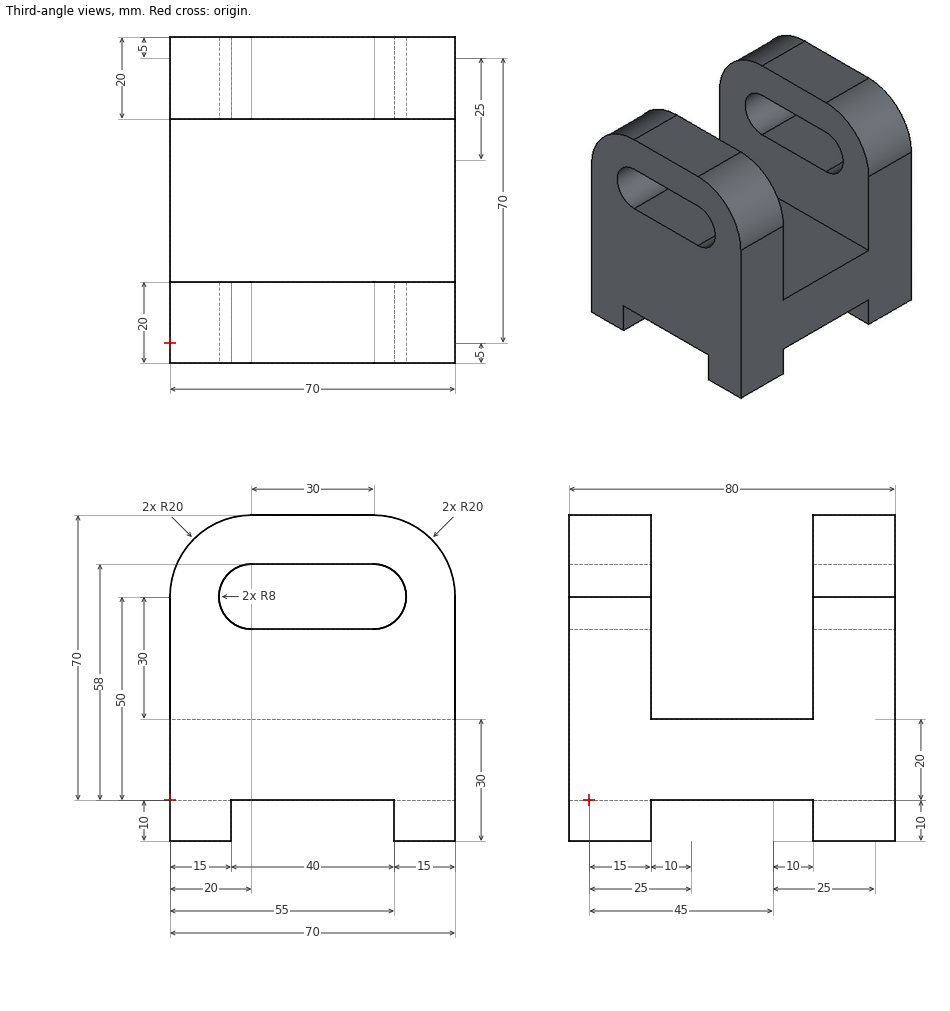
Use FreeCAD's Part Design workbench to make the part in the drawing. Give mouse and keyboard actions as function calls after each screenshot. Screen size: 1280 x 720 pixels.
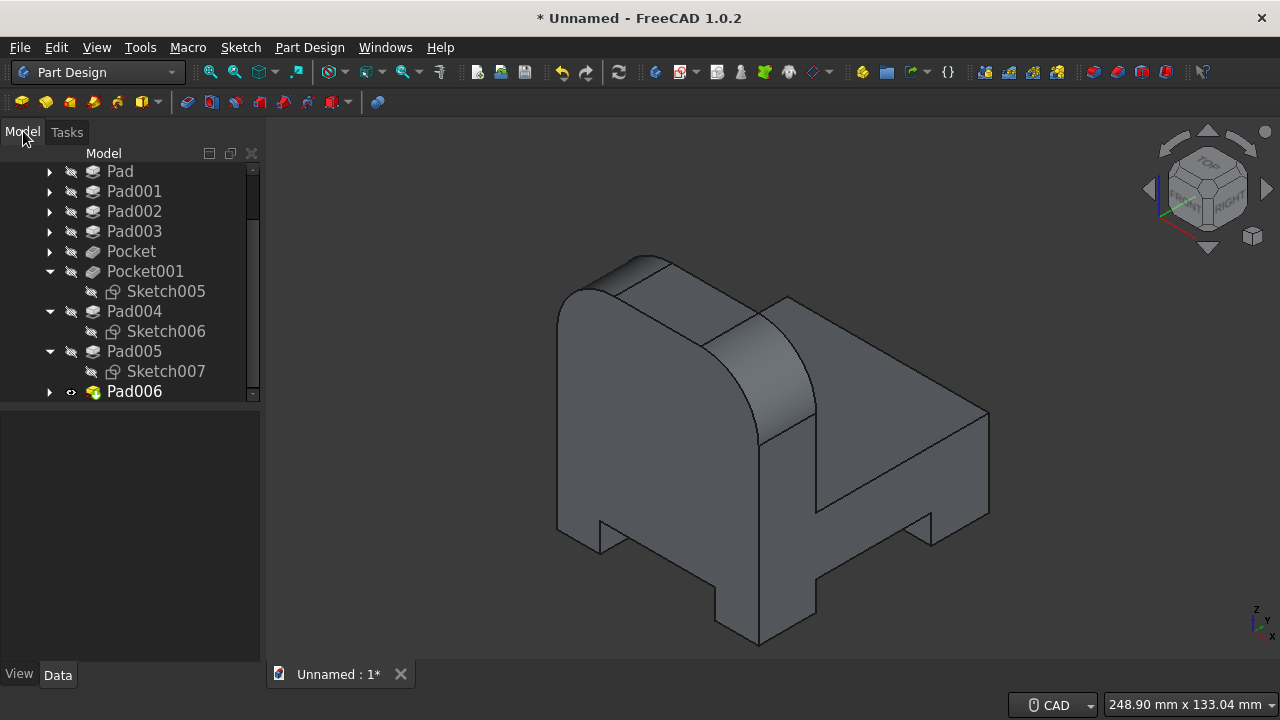
scroll(140, 287, down, 3)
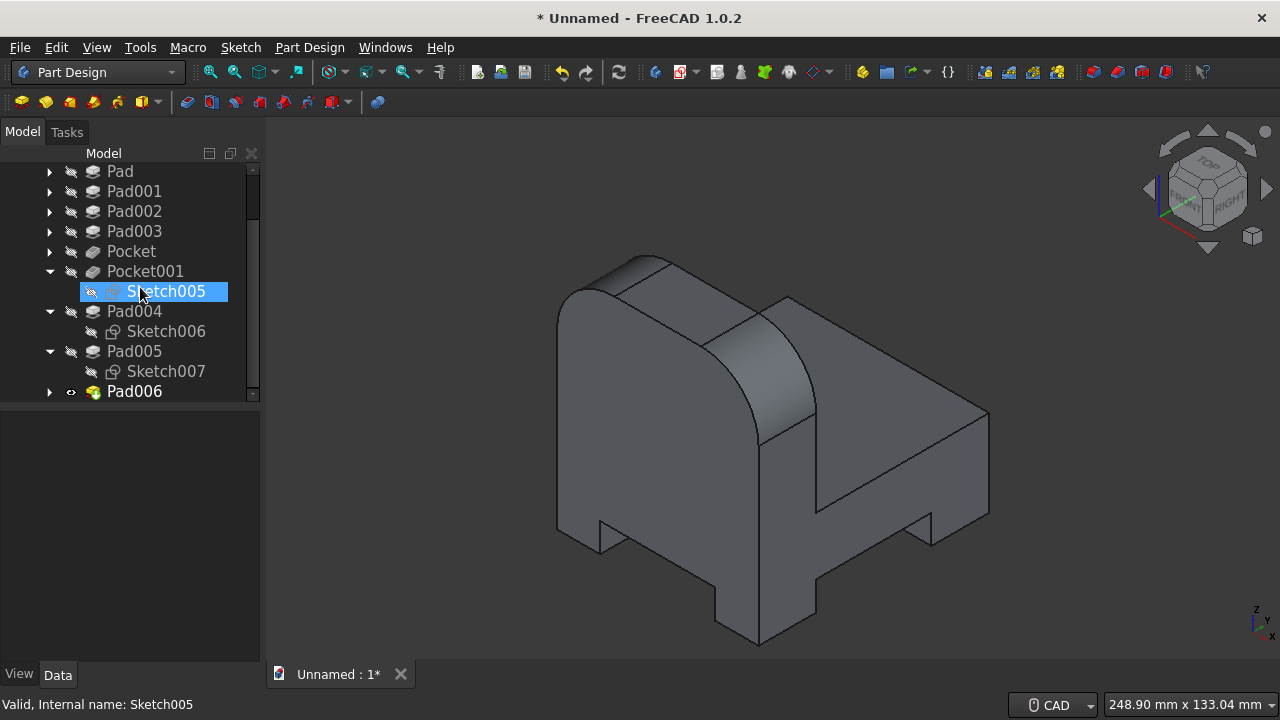
scroll(140, 287, up, 15)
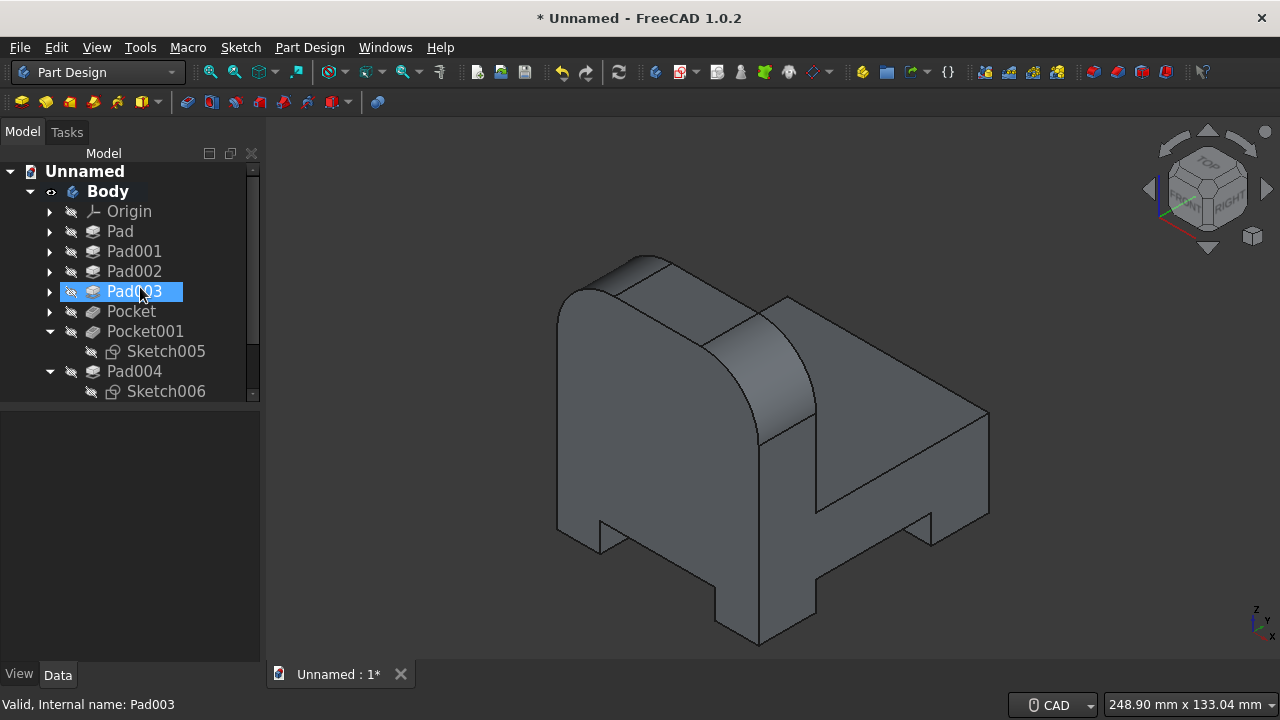
click(50, 212)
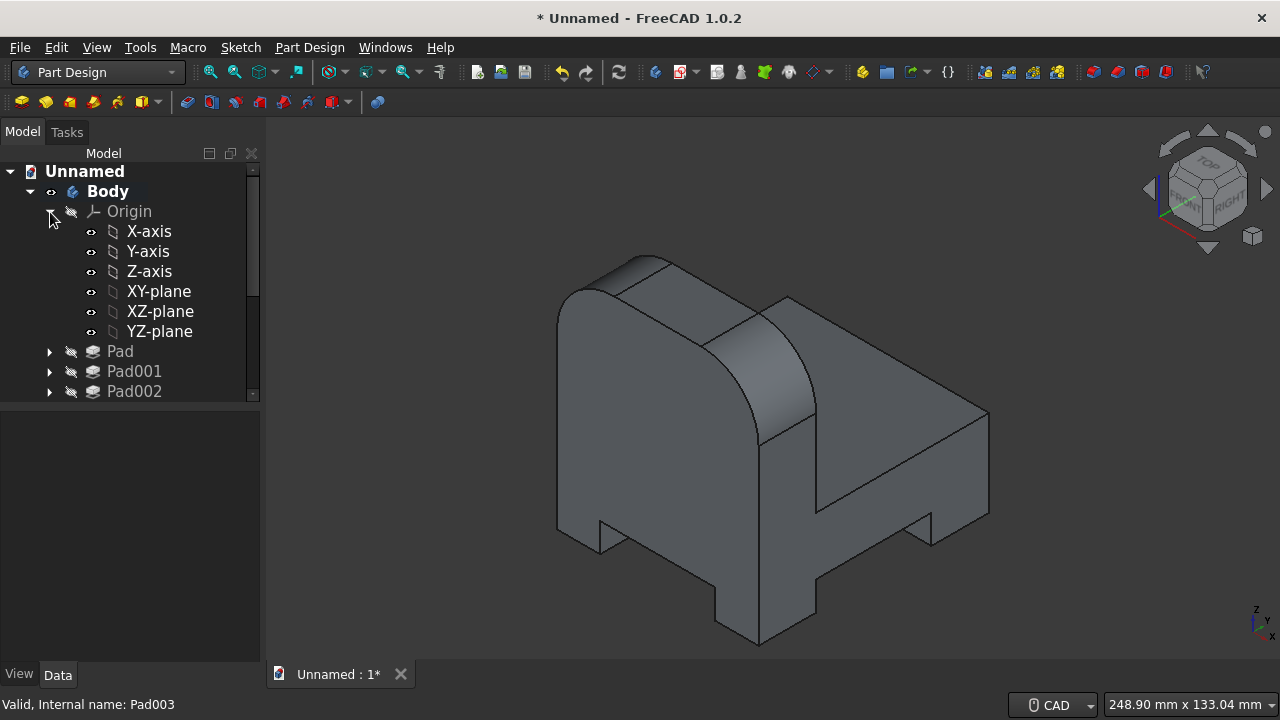
click(136, 312)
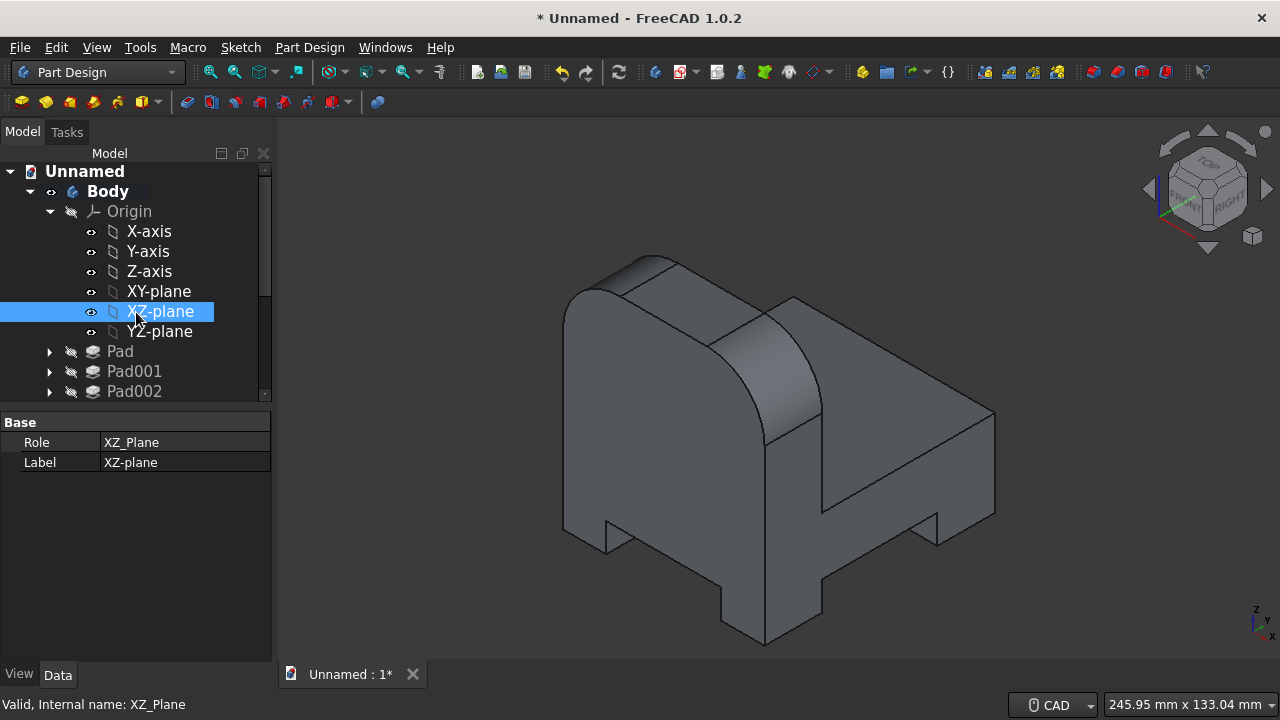
click(814, 72)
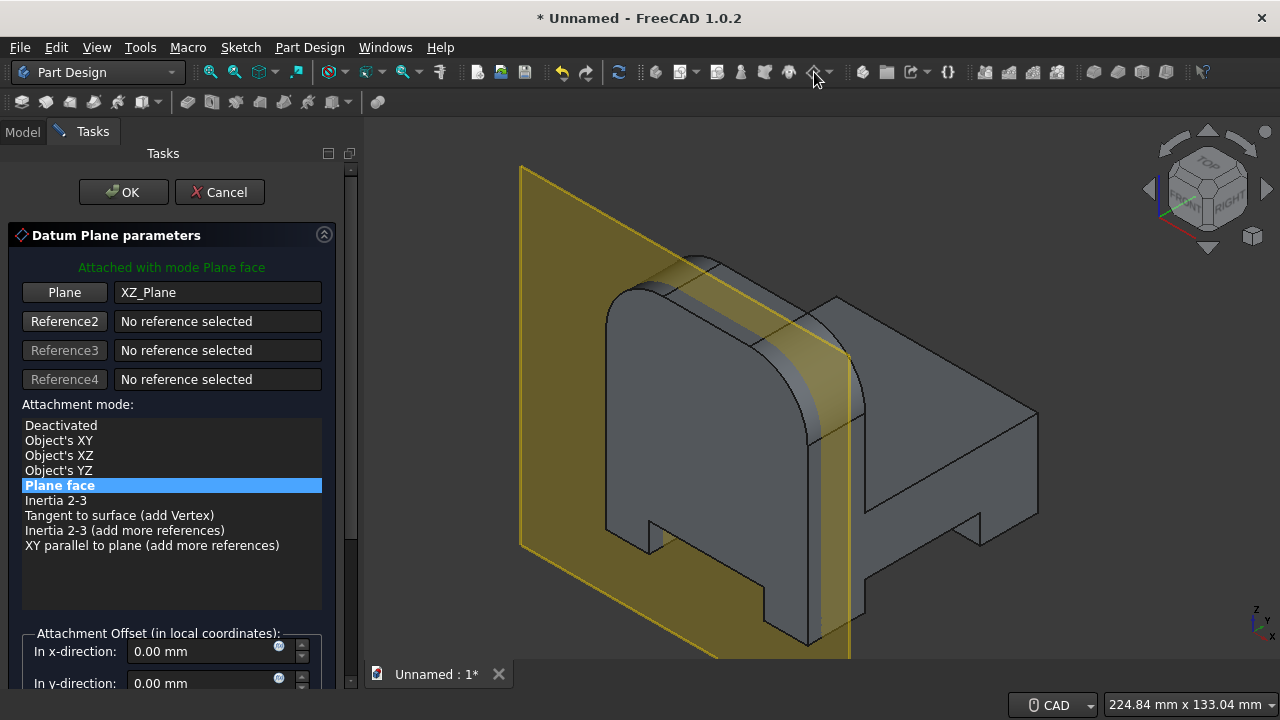
scroll(351, 426, down, 2)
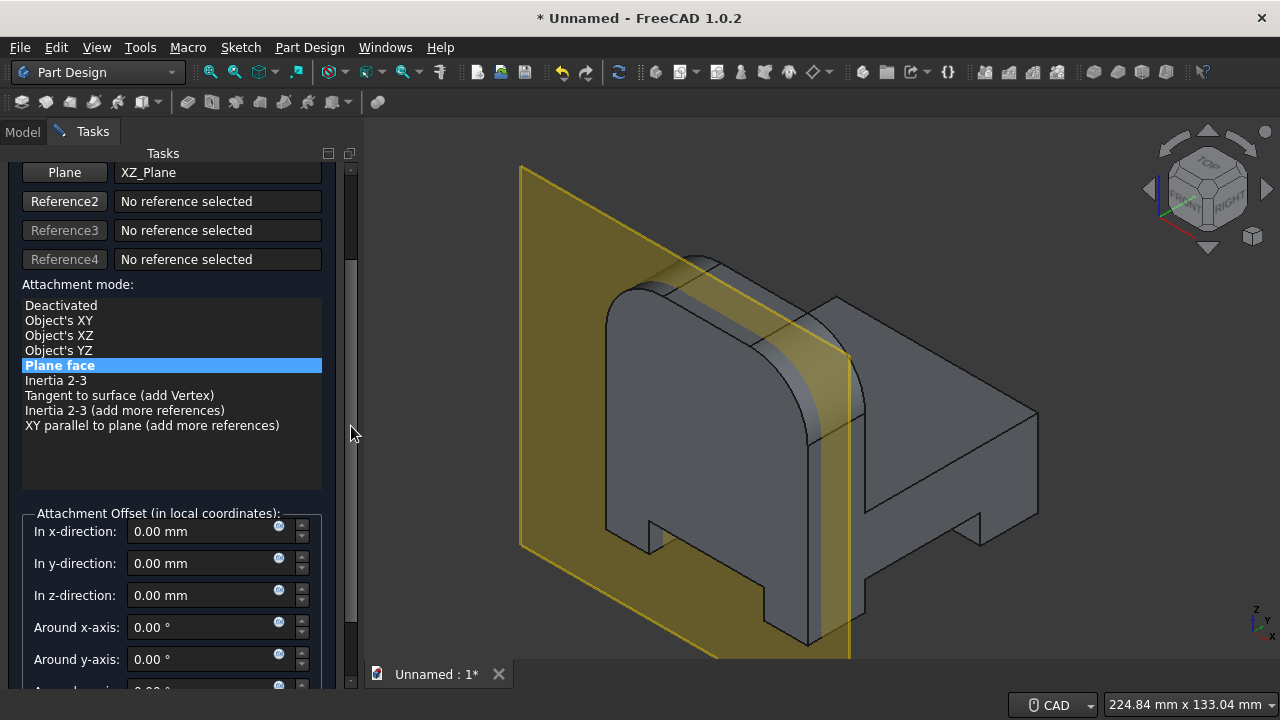
triple_click(210, 595)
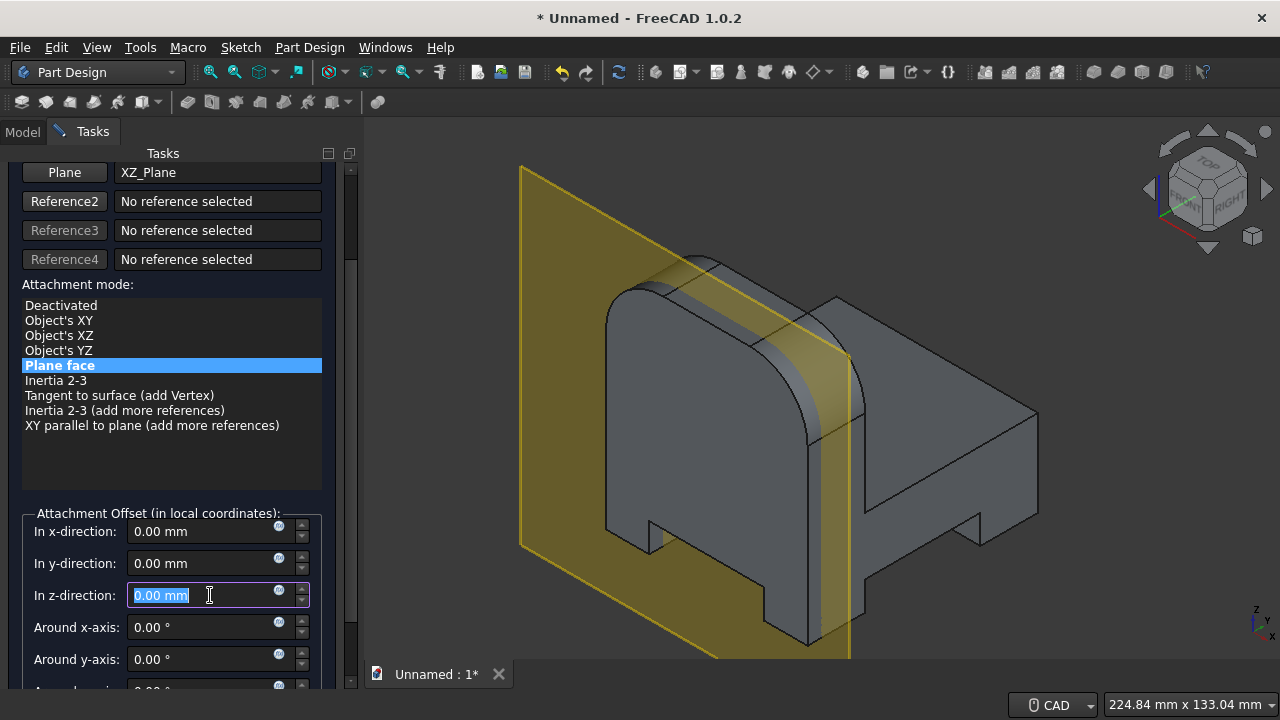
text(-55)
key(Tab)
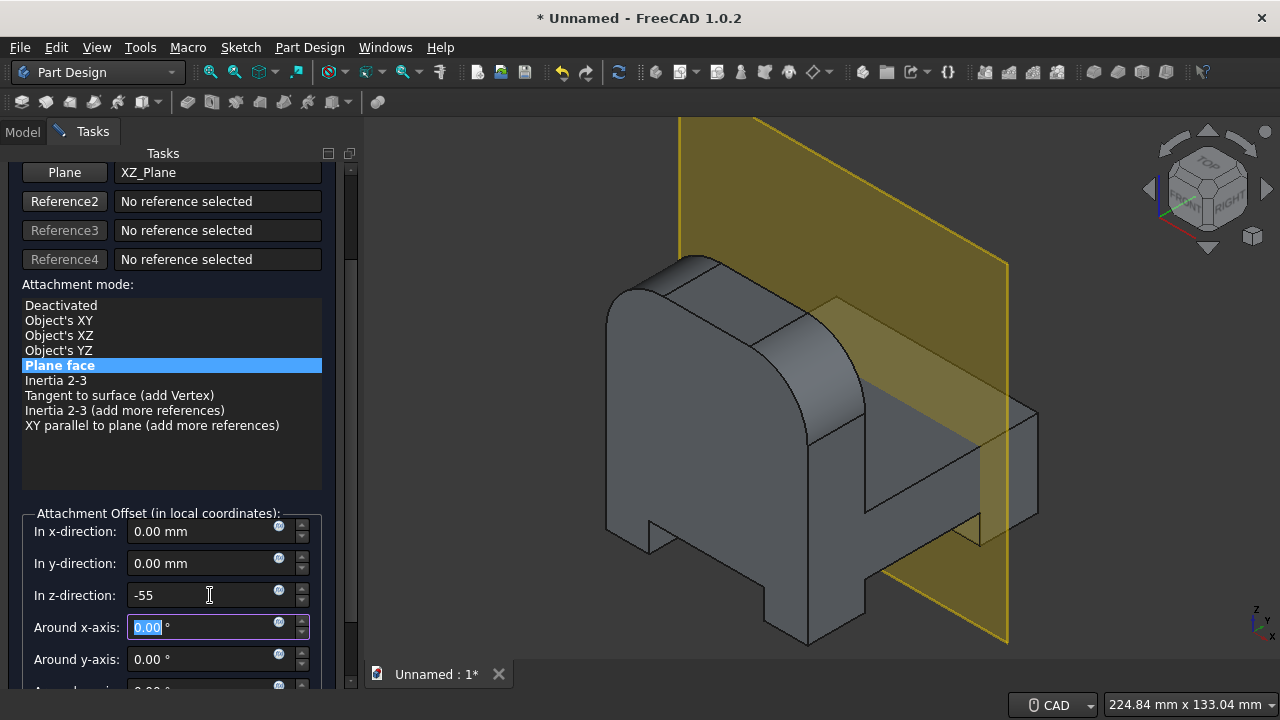
scroll(351, 426, up, 3)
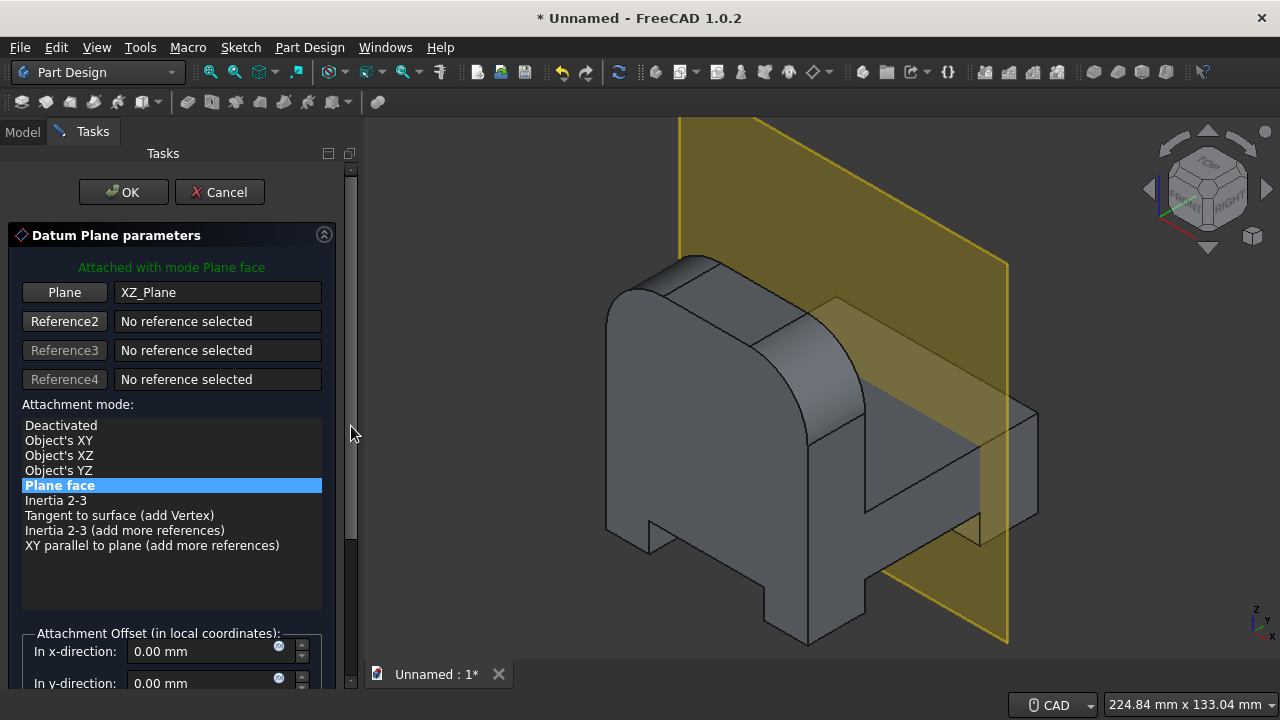
click(124, 192)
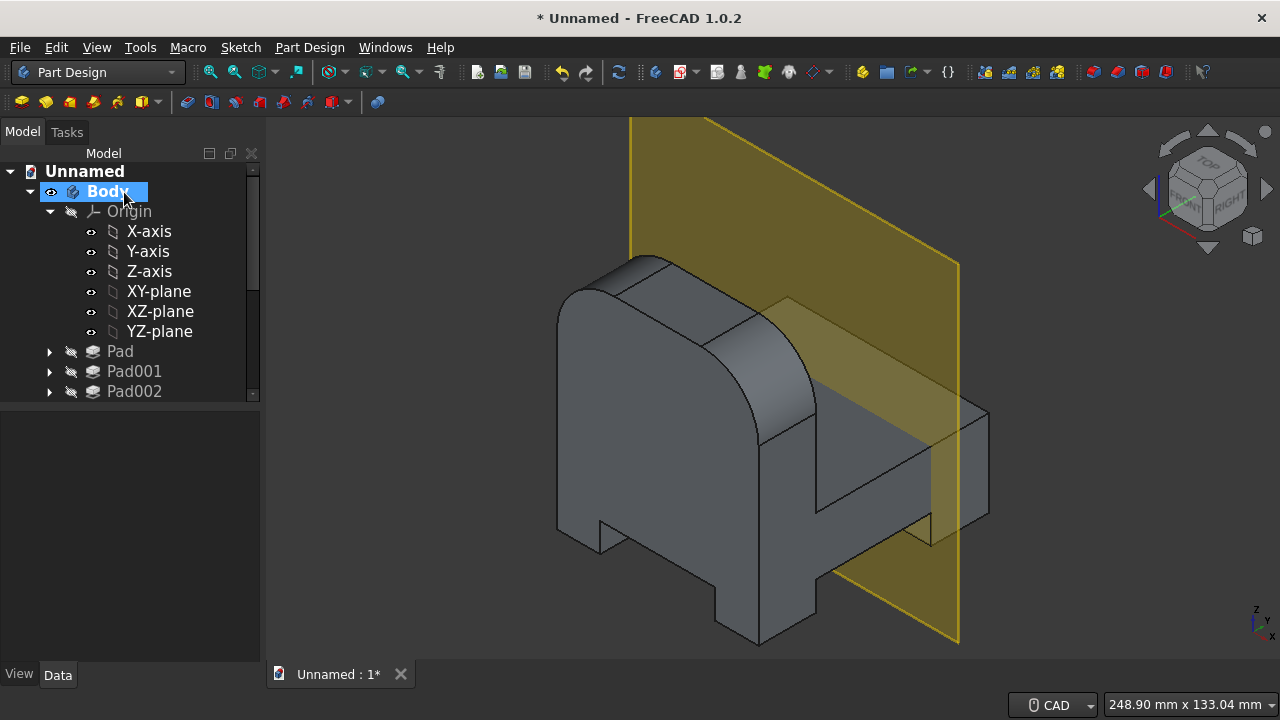
scroll(100, 287, down, 3)